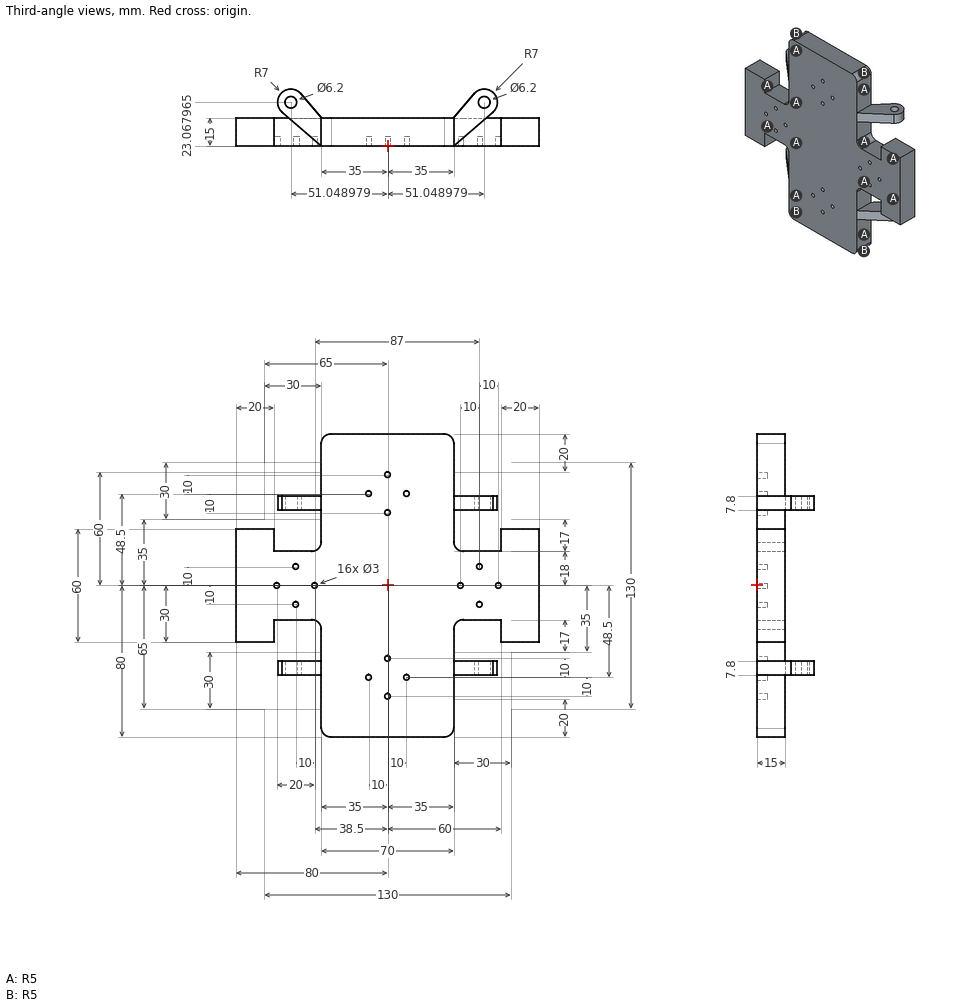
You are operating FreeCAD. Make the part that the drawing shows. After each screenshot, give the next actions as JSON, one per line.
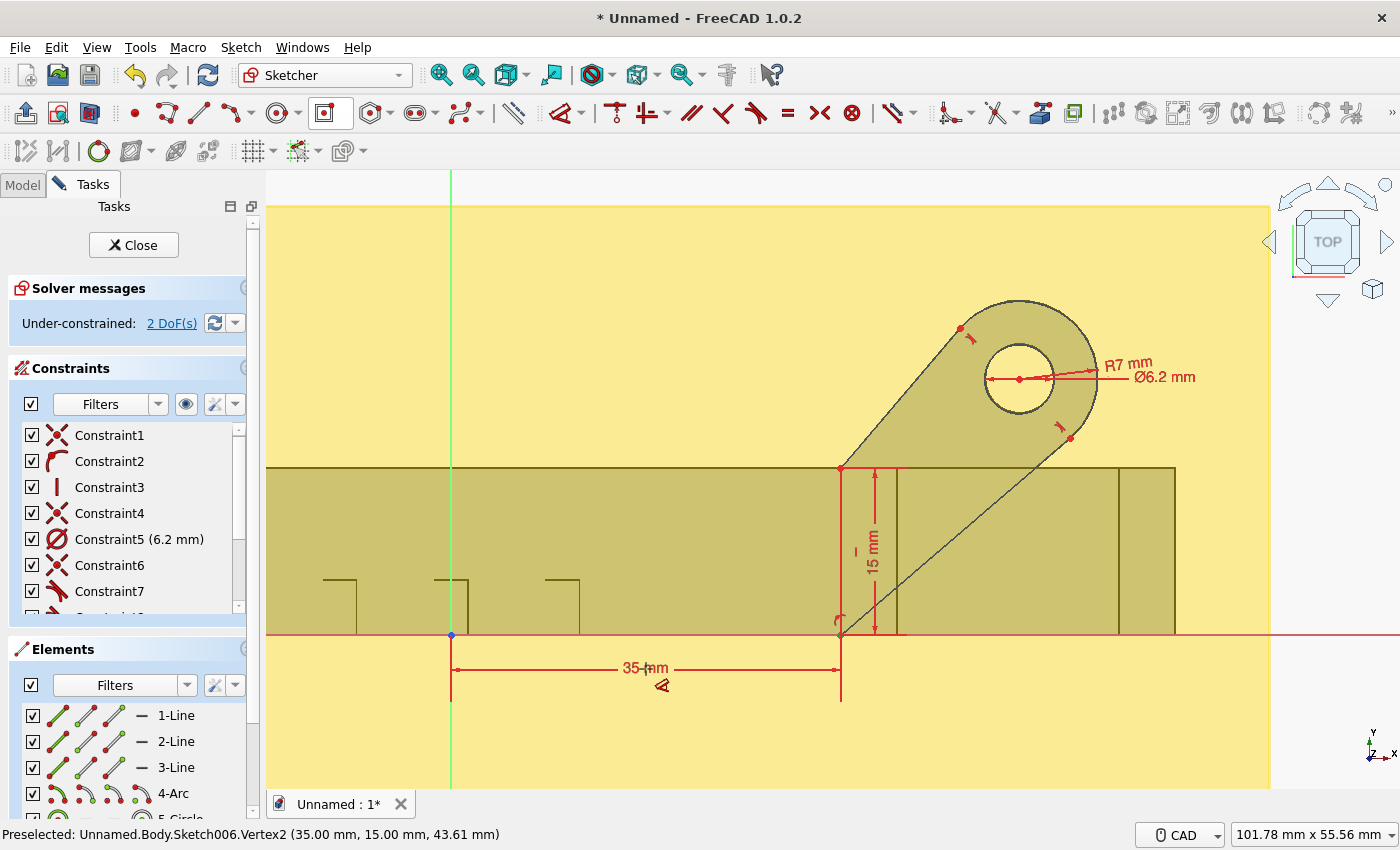
{"action": "left_click", "coordinate": [1019, 379]}
{"action": "left_click", "coordinate": [735, 669]}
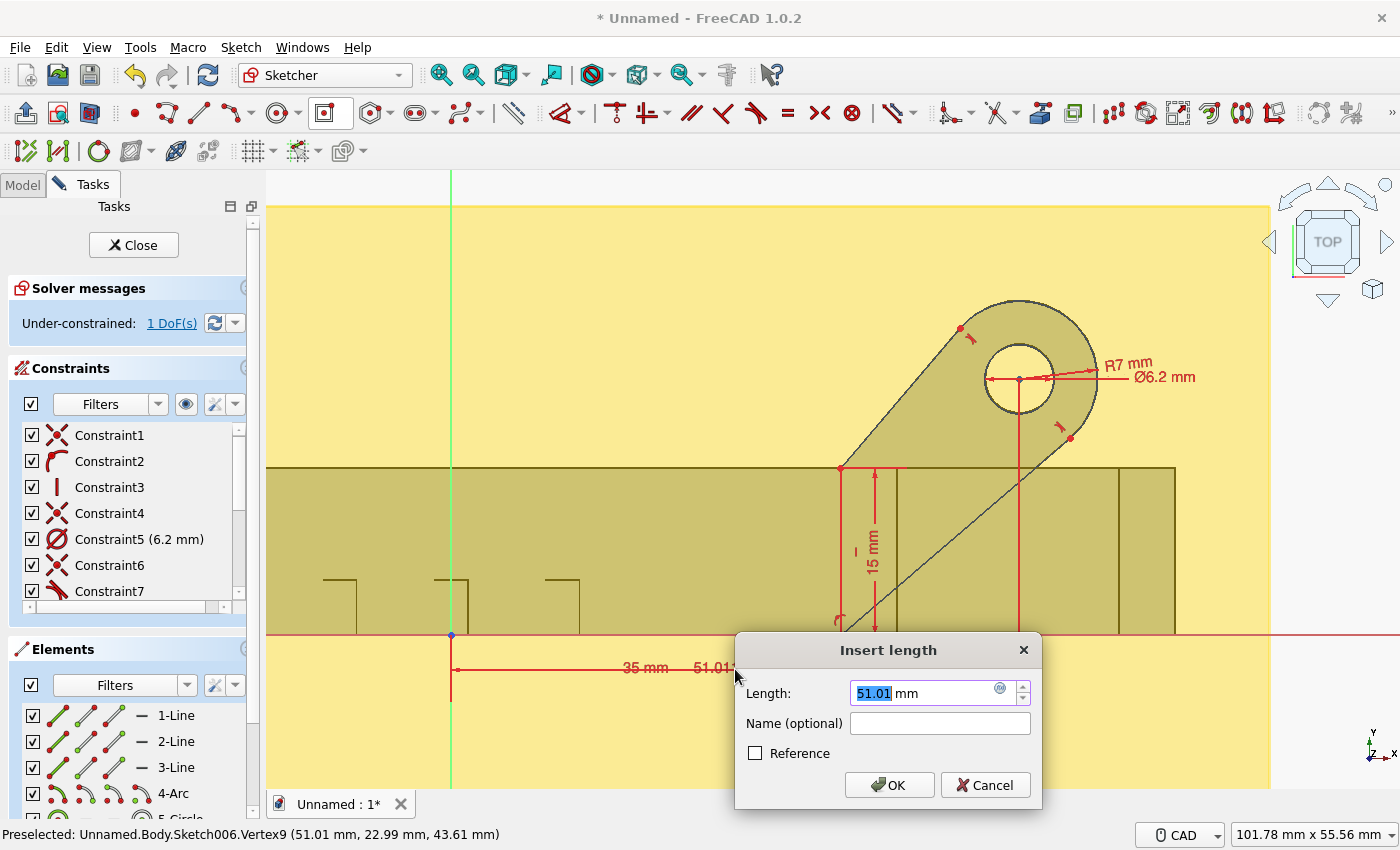
{"action": "type", "text": "51.048979"}
{"action": "key", "text": "Return"}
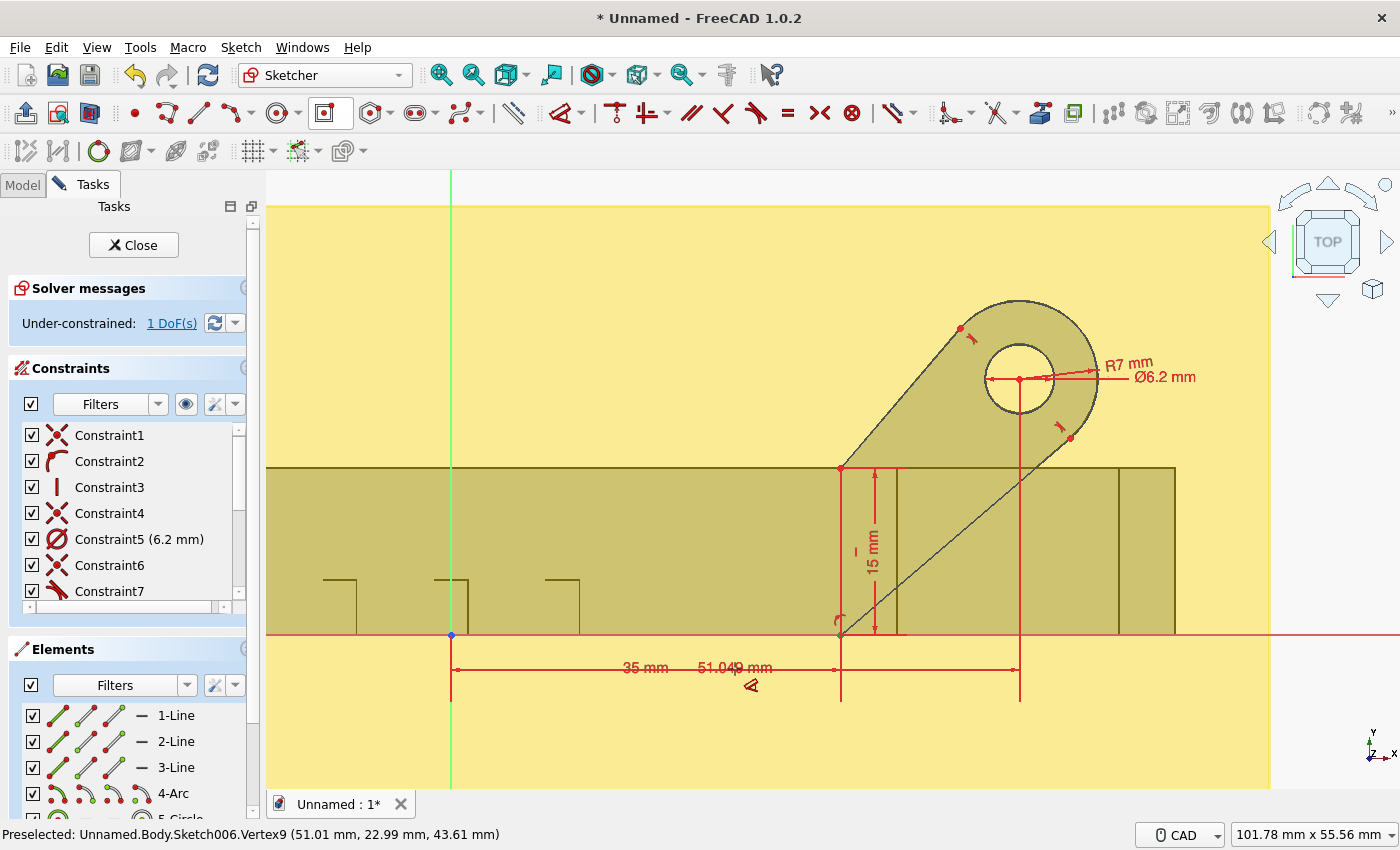
{"action": "left_click", "coordinate": [1020, 379]}
{"action": "left_click", "coordinate": [417, 507]}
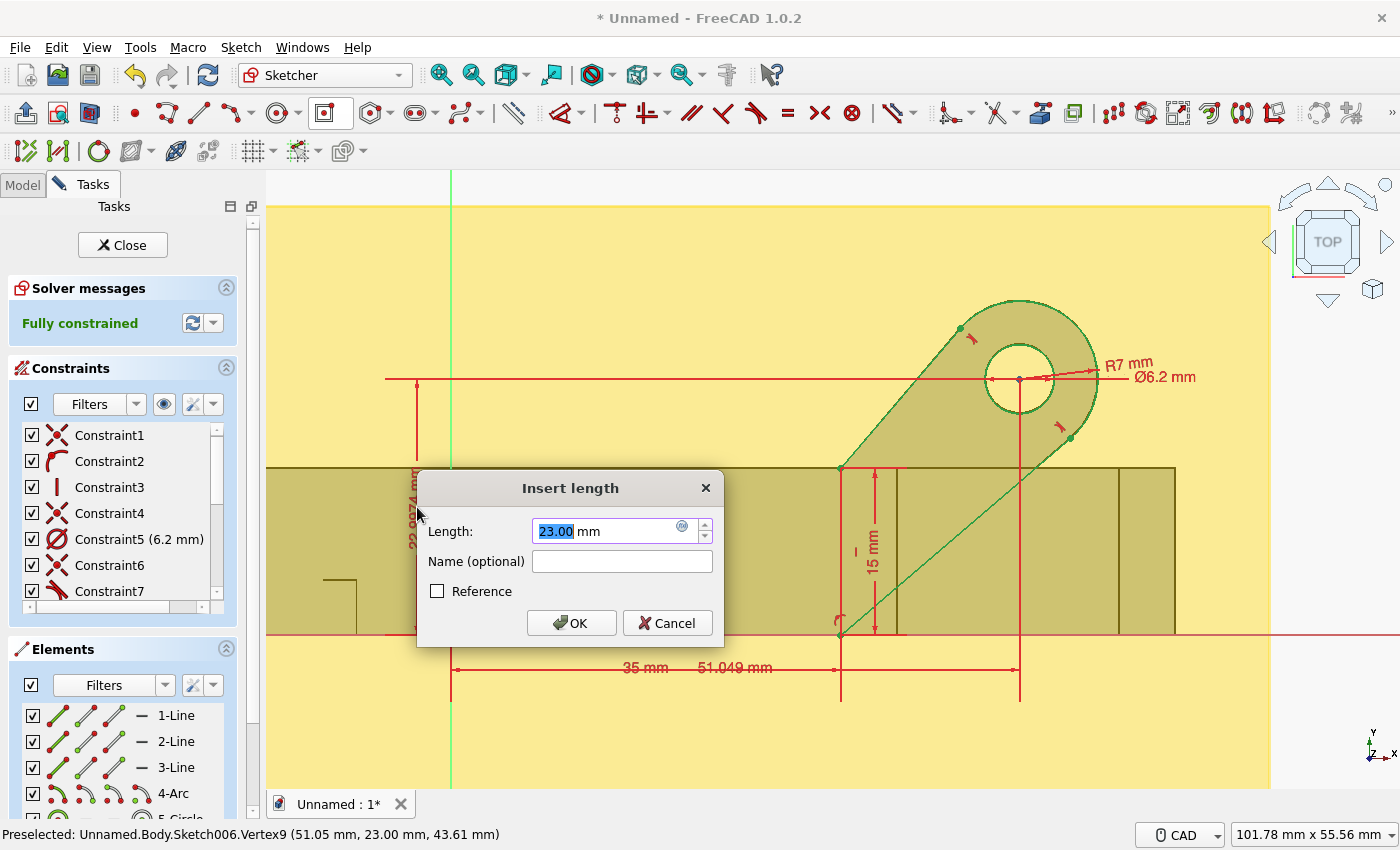
{"action": "type", "text": "23.067965"}
{"action": "key", "text": "Return"}
{"action": "key", "text": "Escape"}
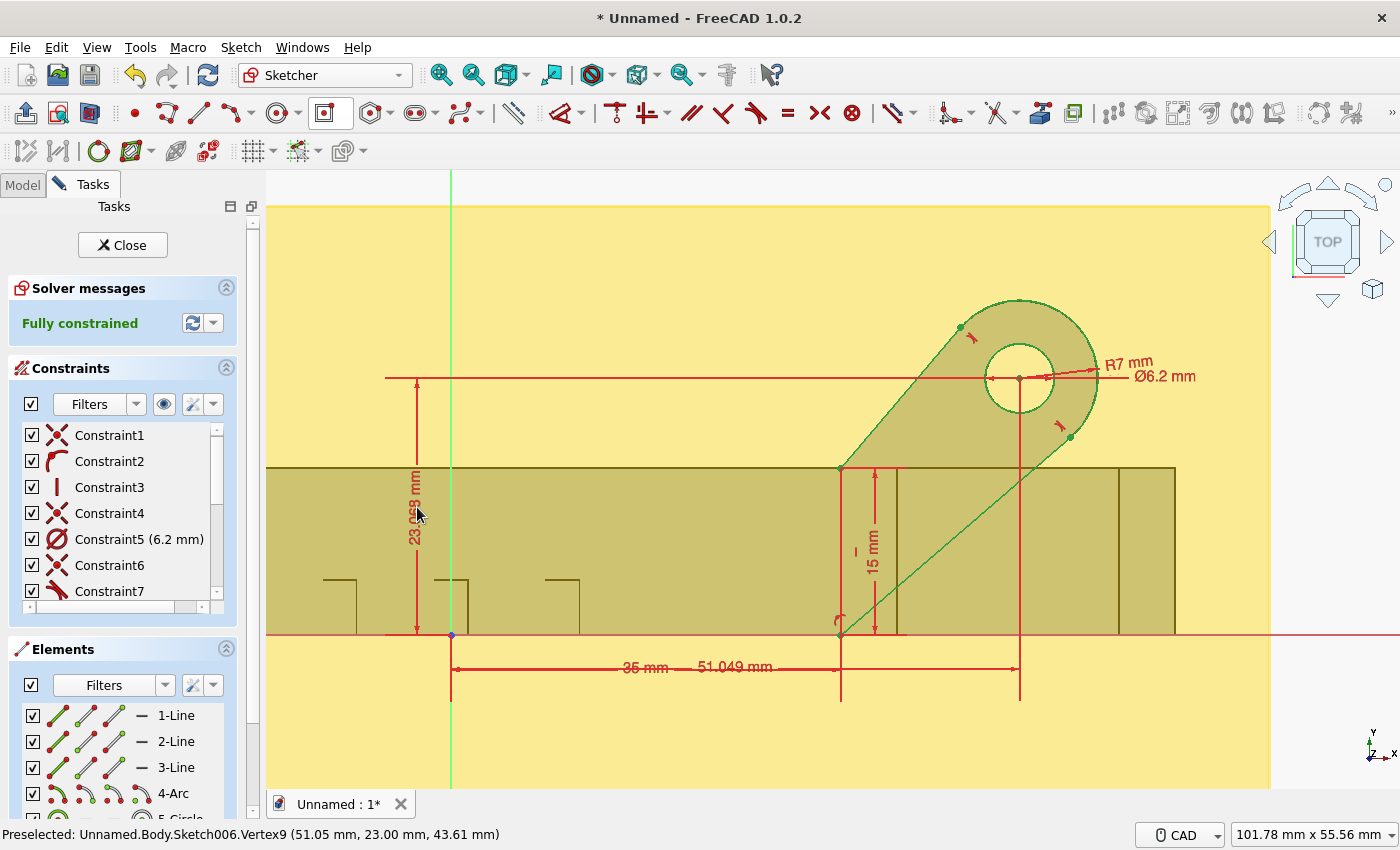
{"action": "left_click", "coordinate": [123, 245]}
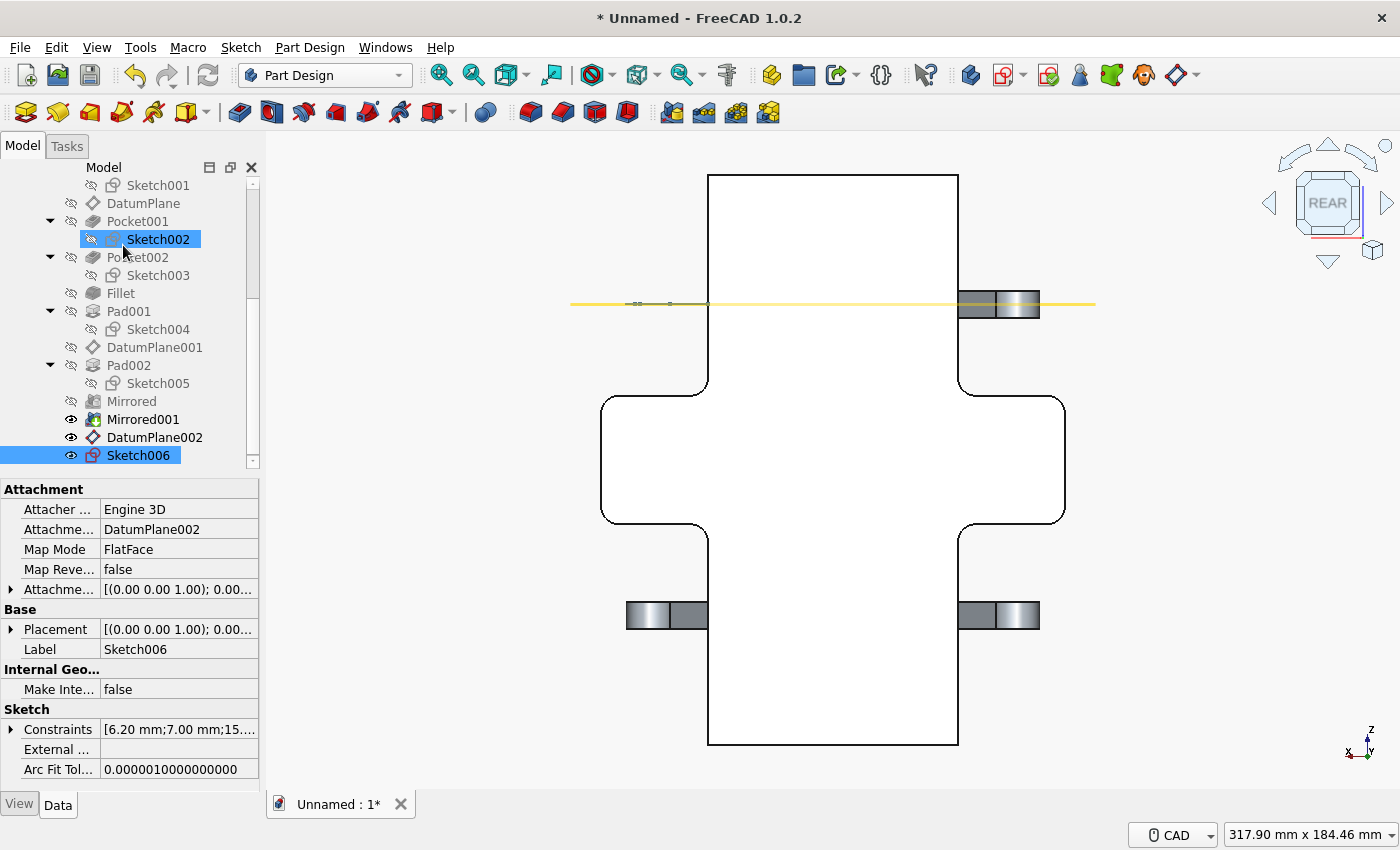
{"action": "left_click", "coordinate": [26, 112]}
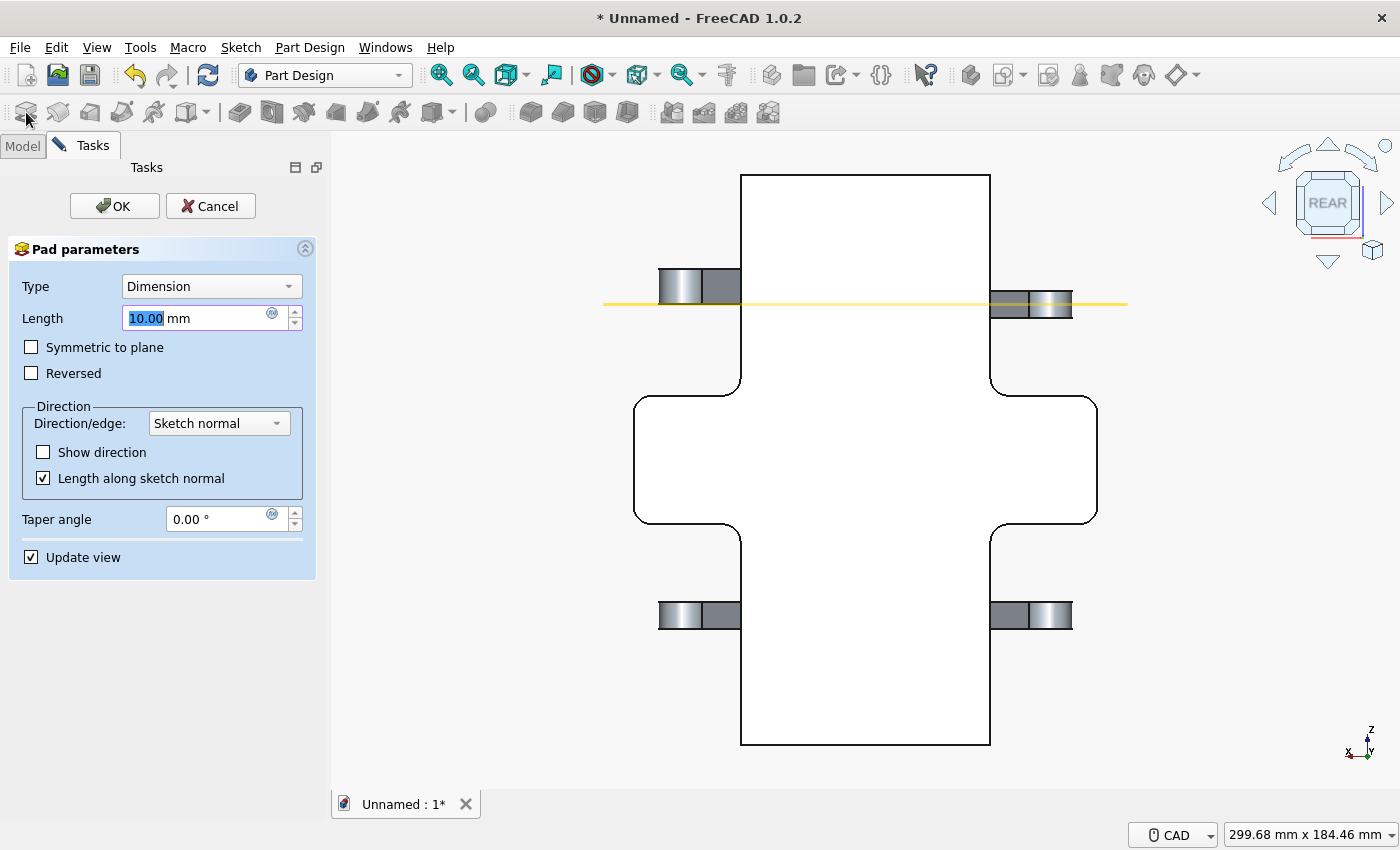
{"action": "type", "text": "7.8"}
{"action": "key", "text": "Tab"}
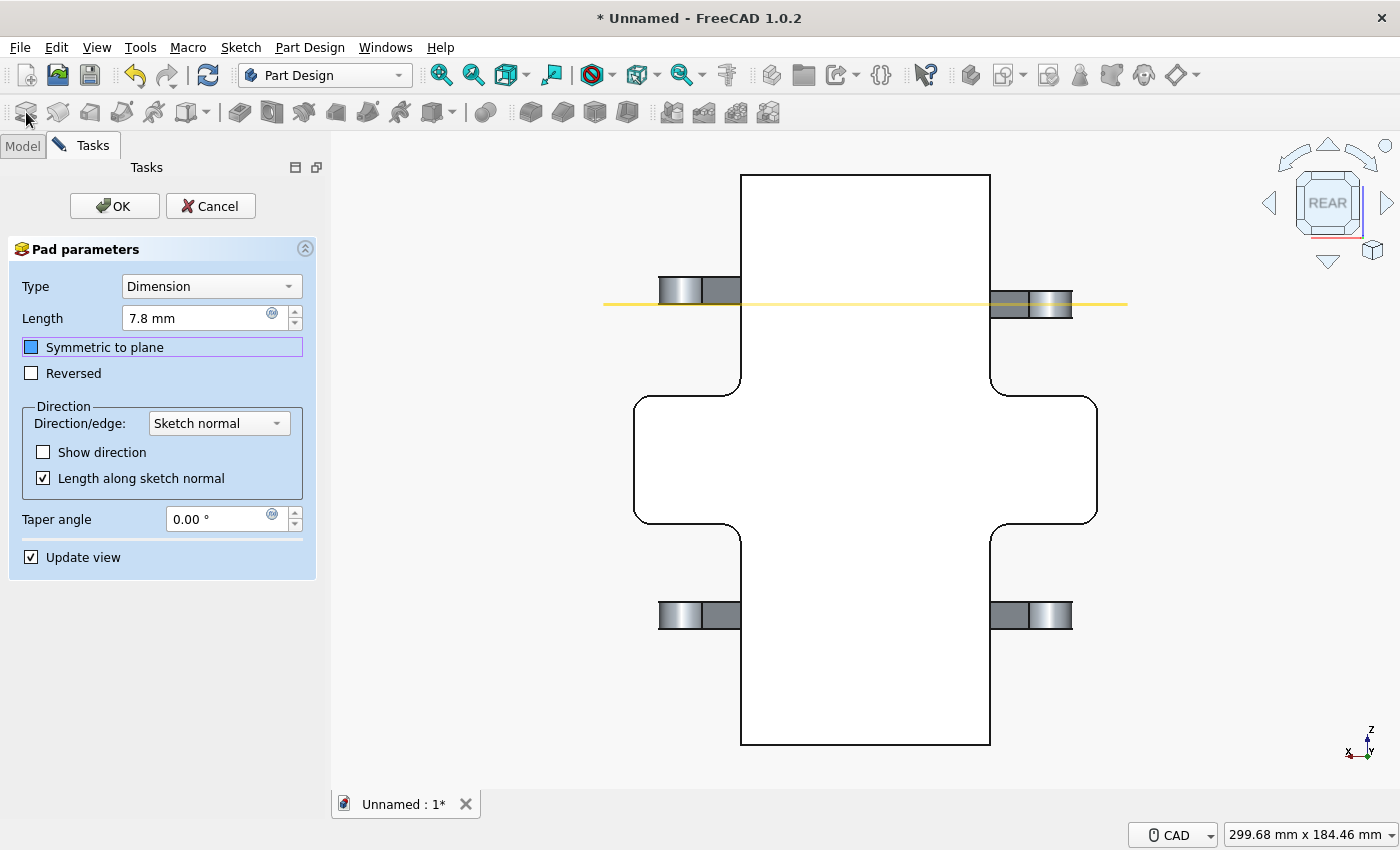
{"action": "left_click", "coordinate": [30, 347]}